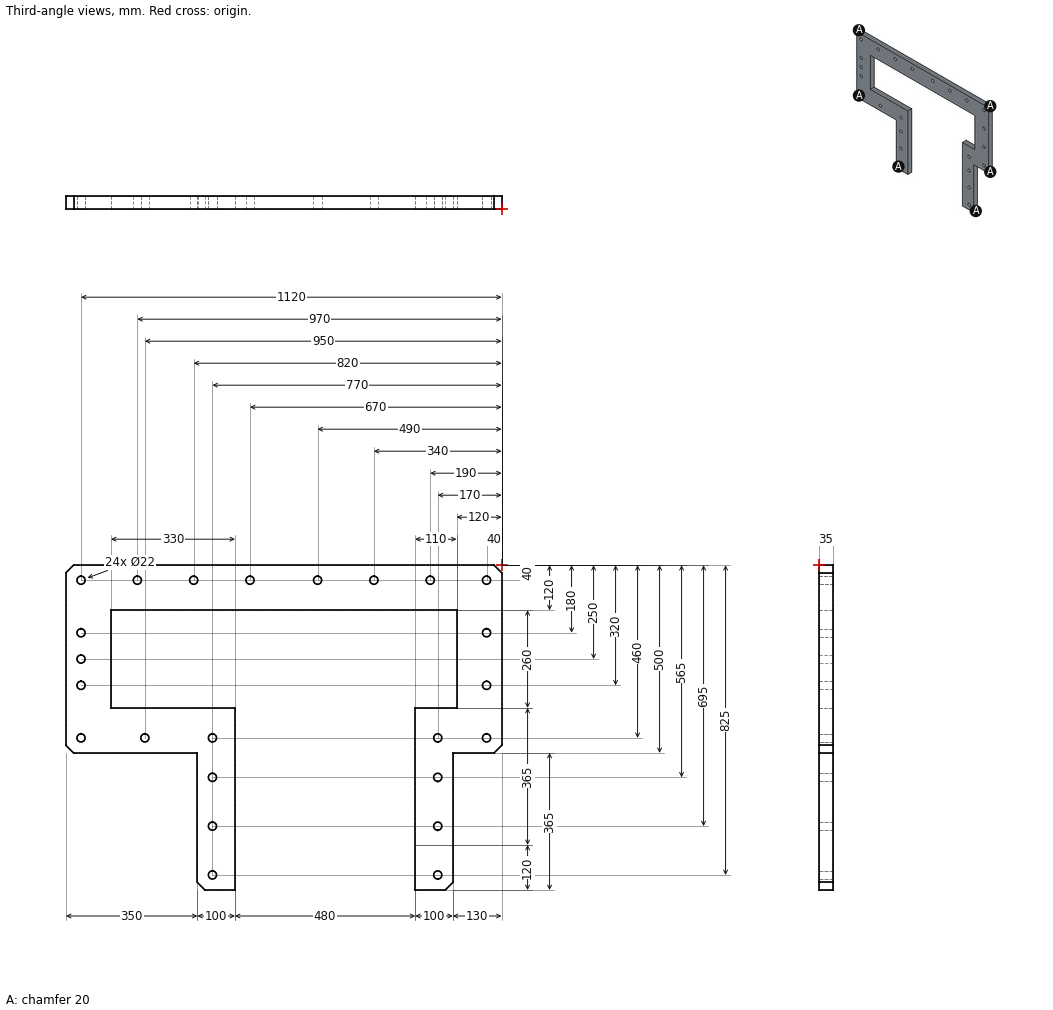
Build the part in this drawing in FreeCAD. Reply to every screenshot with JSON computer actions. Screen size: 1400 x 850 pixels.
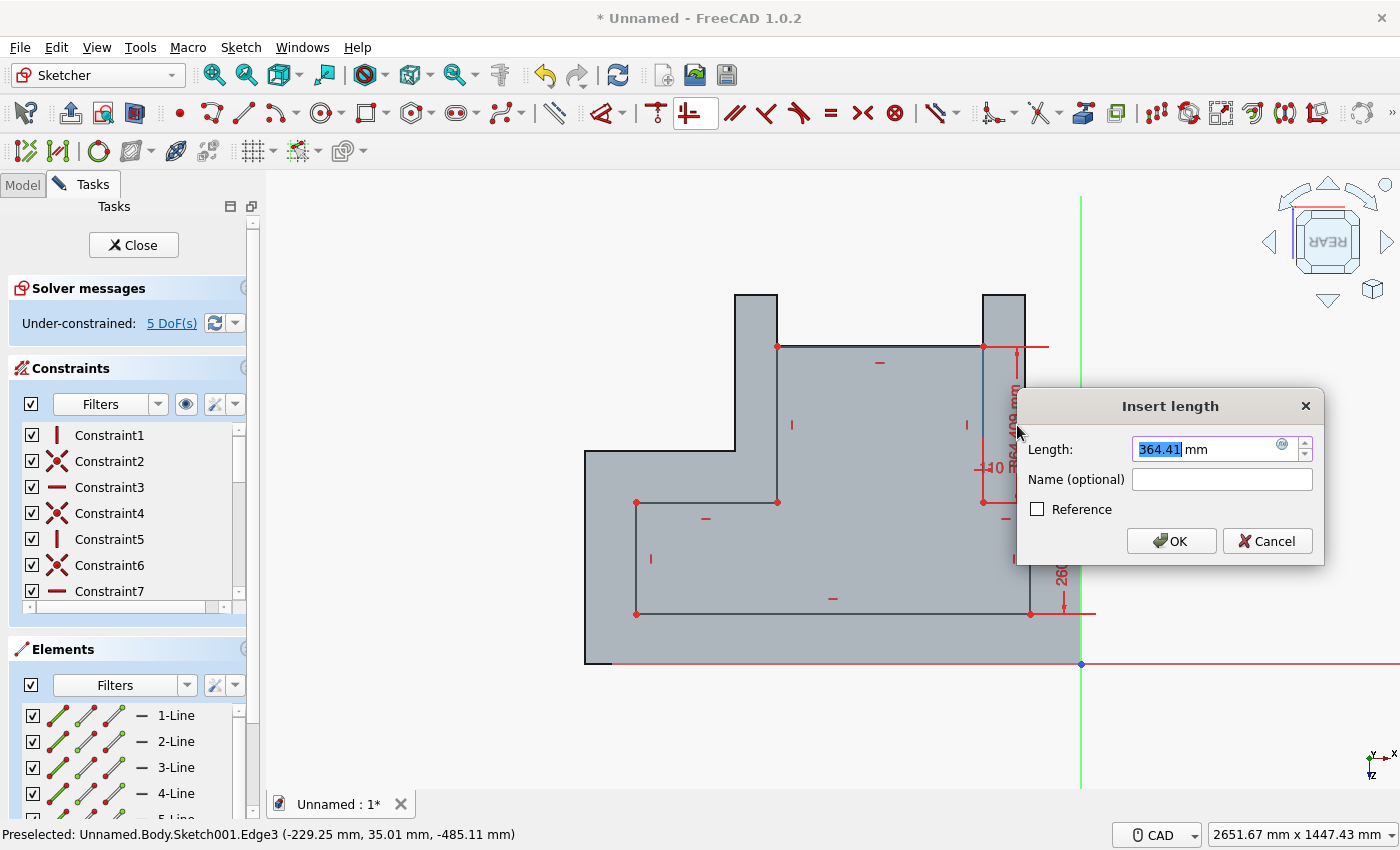
{"action": "type", "text": "365"}
{"action": "key", "text": "Return"}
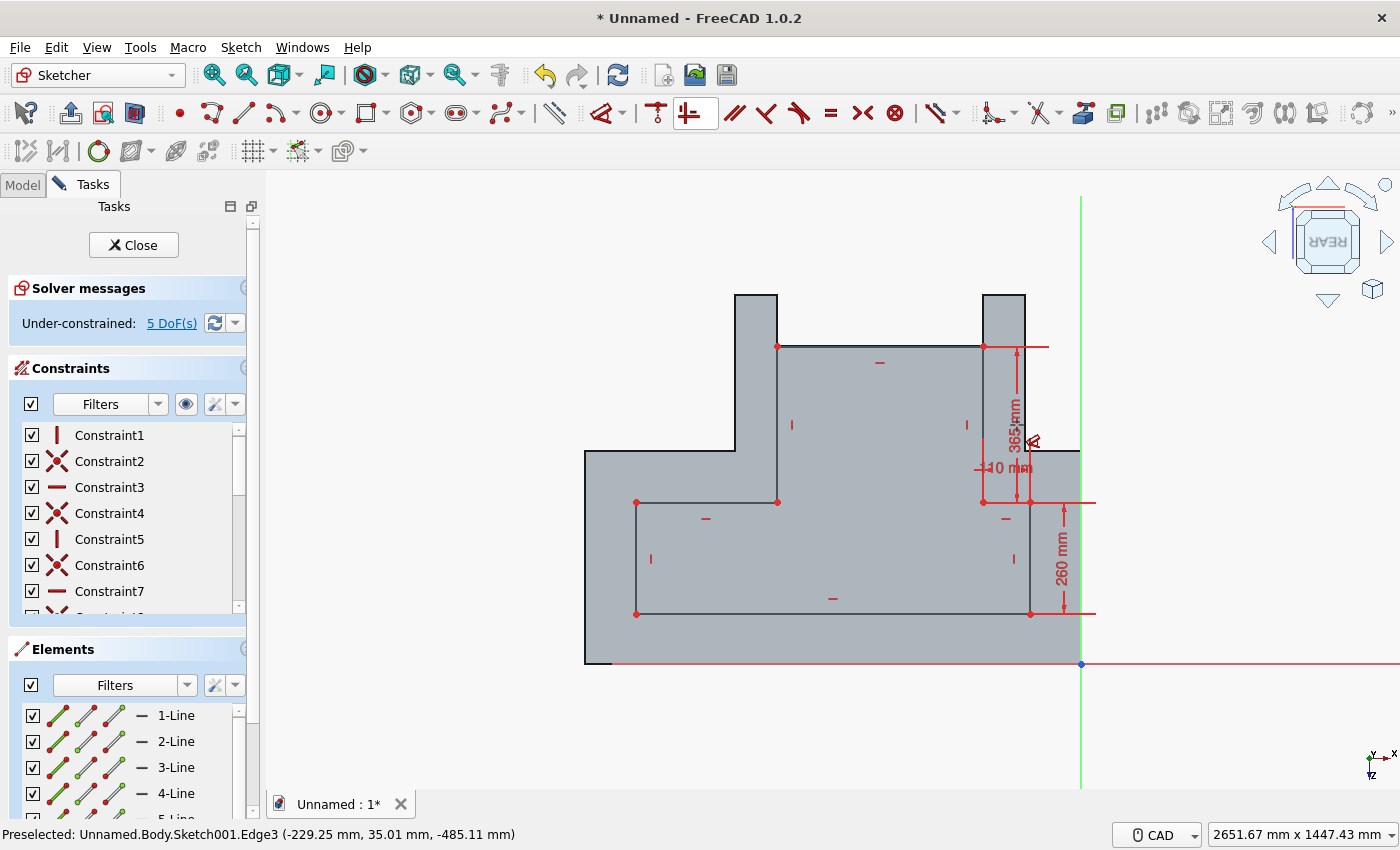
{"action": "left_click", "coordinate": [921, 347]}
{"action": "left_click", "coordinate": [880, 313]}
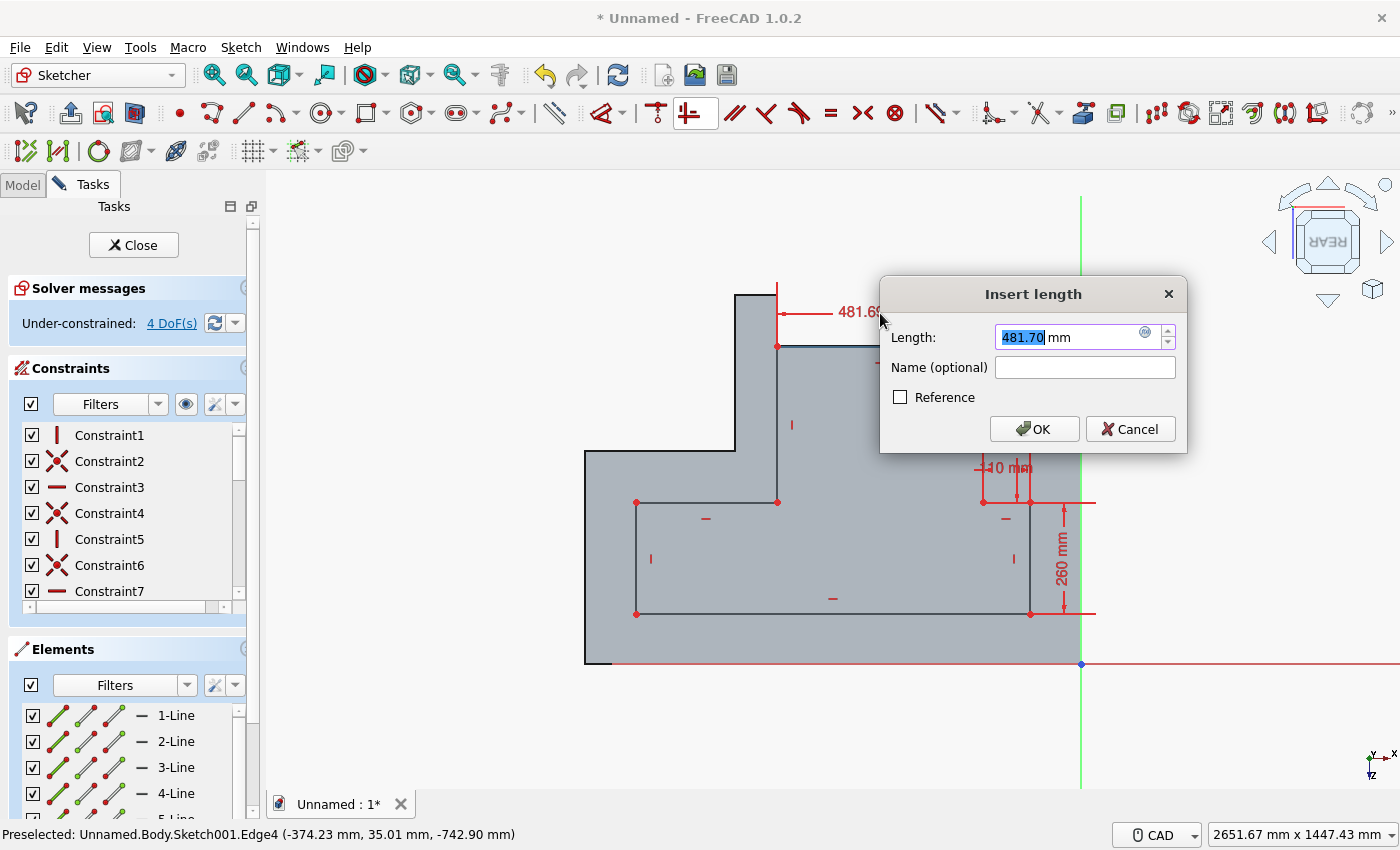
{"action": "type", "text": "480"}
{"action": "key", "text": "Return"}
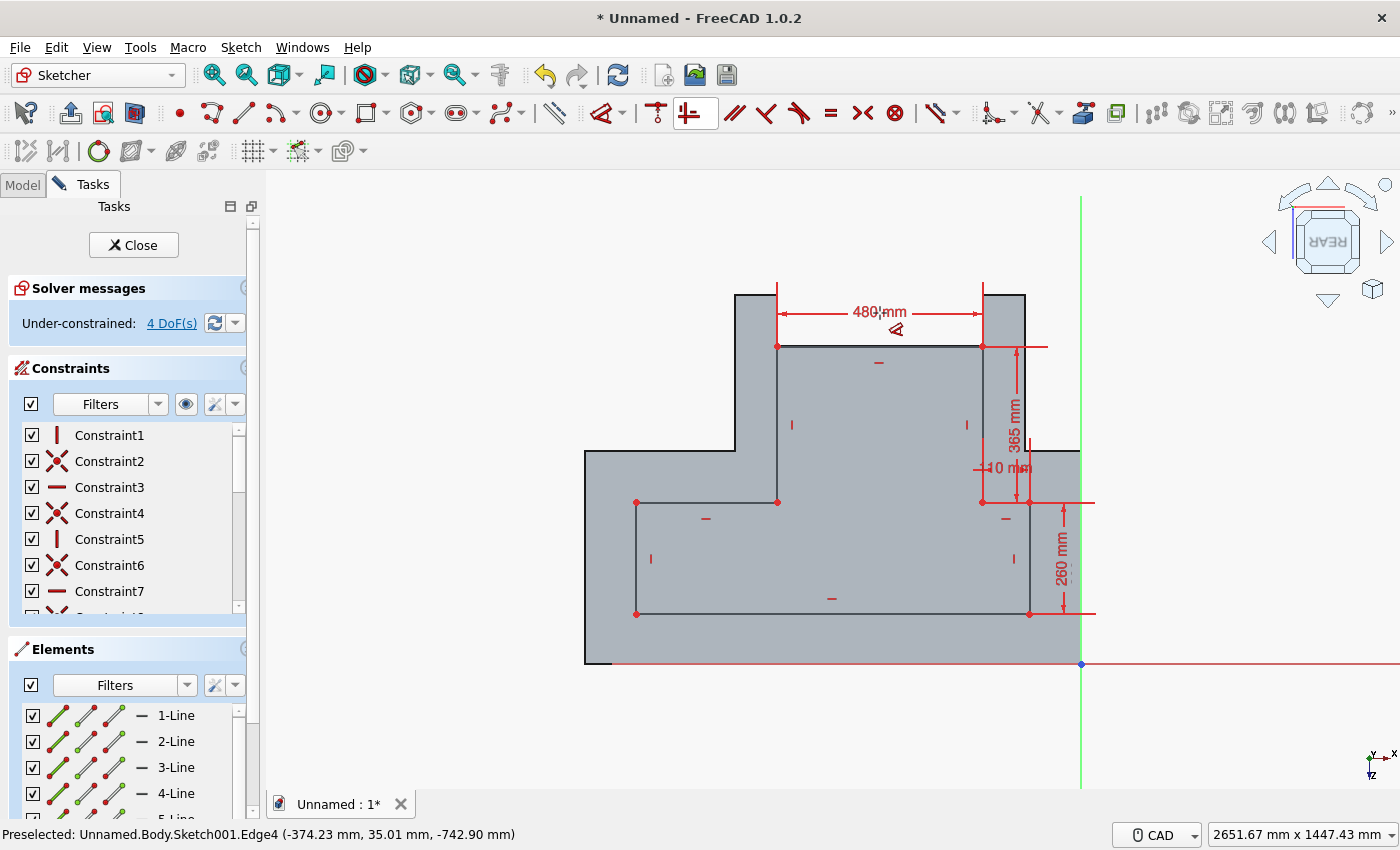
{"action": "left_click", "coordinate": [777, 394]}
{"action": "left_click", "coordinate": [743, 425]}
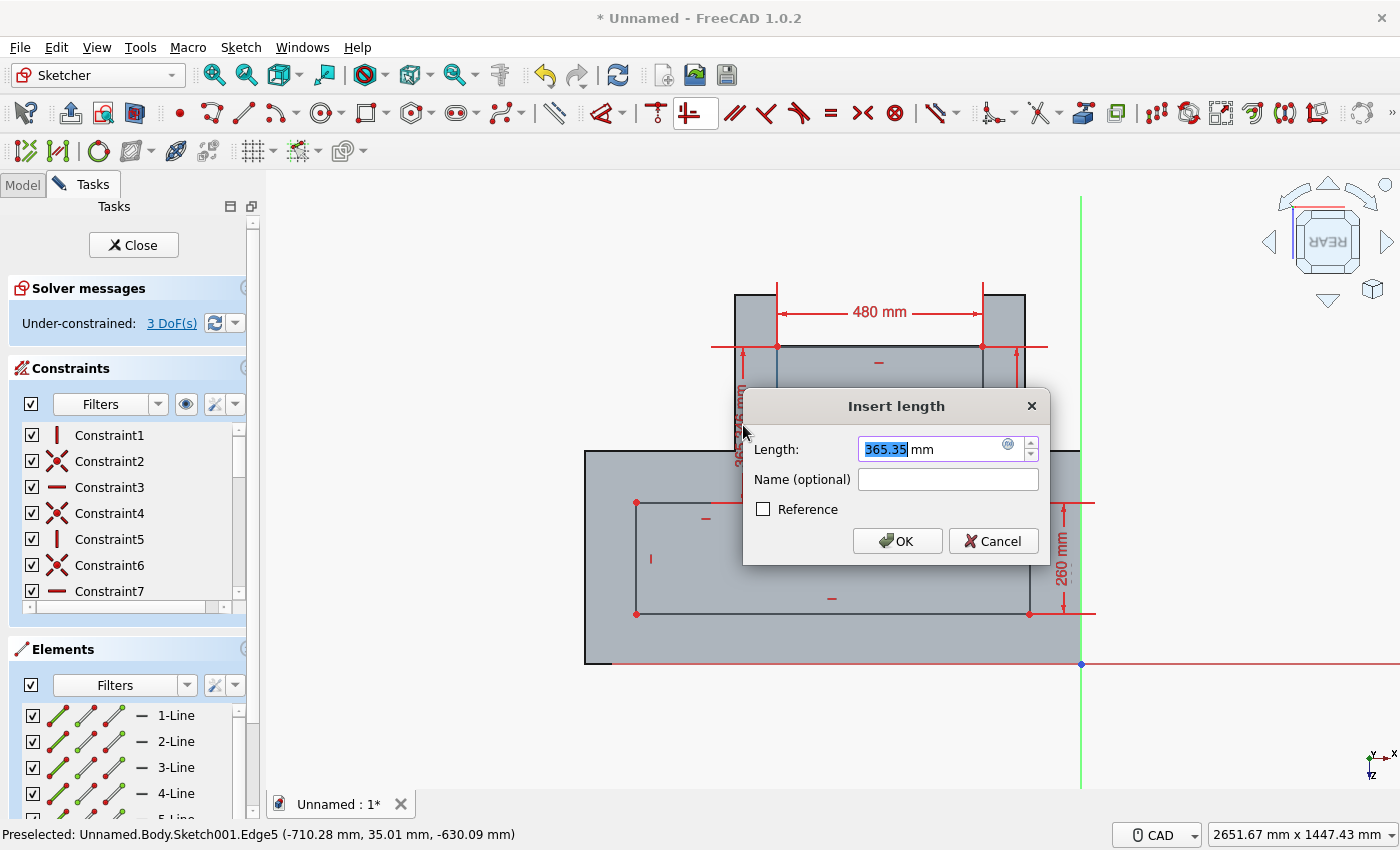
{"action": "type", "text": "365"}
{"action": "key", "text": "Return"}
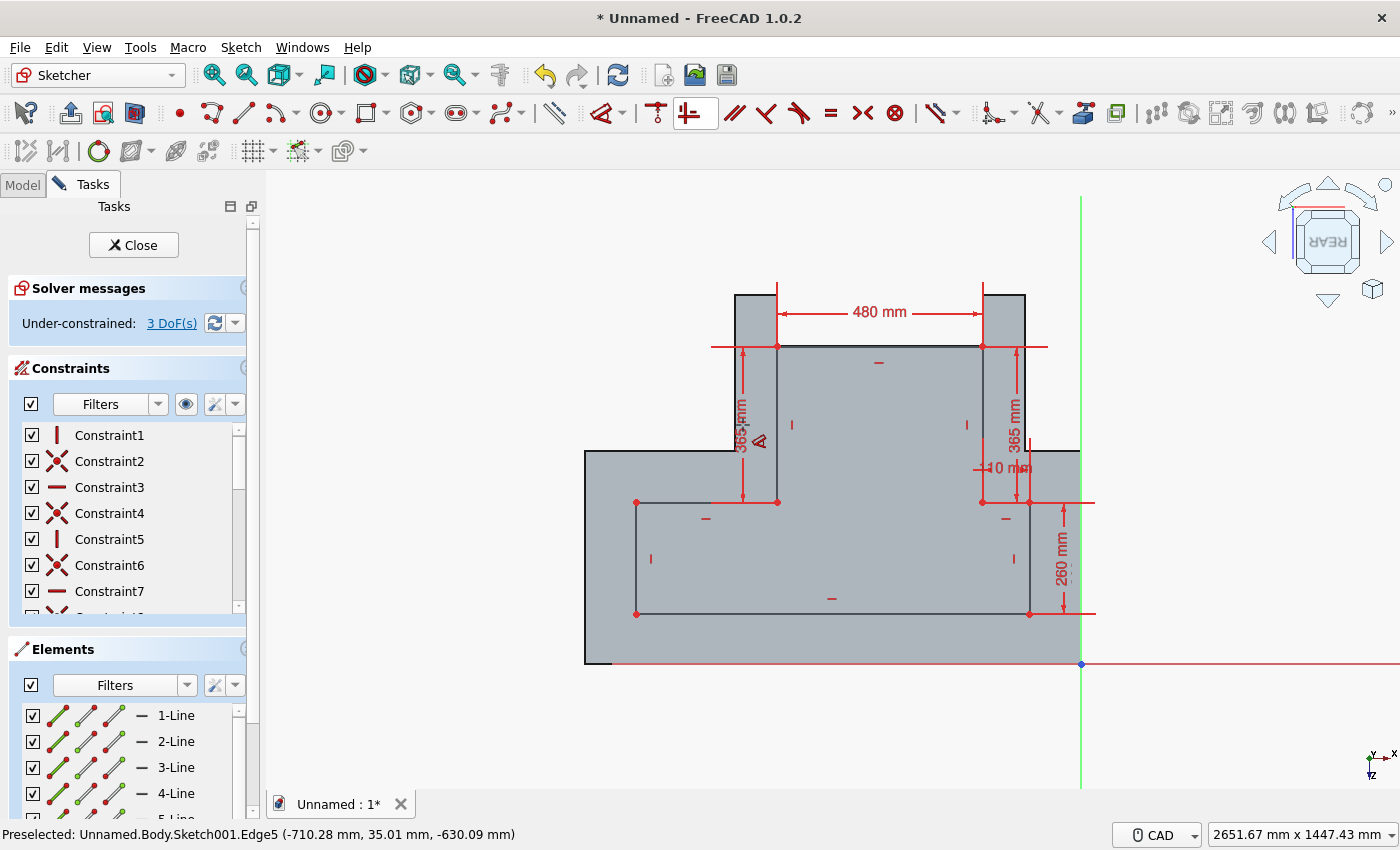
{"action": "left_click", "coordinate": [735, 503]}
{"action": "left_click", "coordinate": [707, 469]}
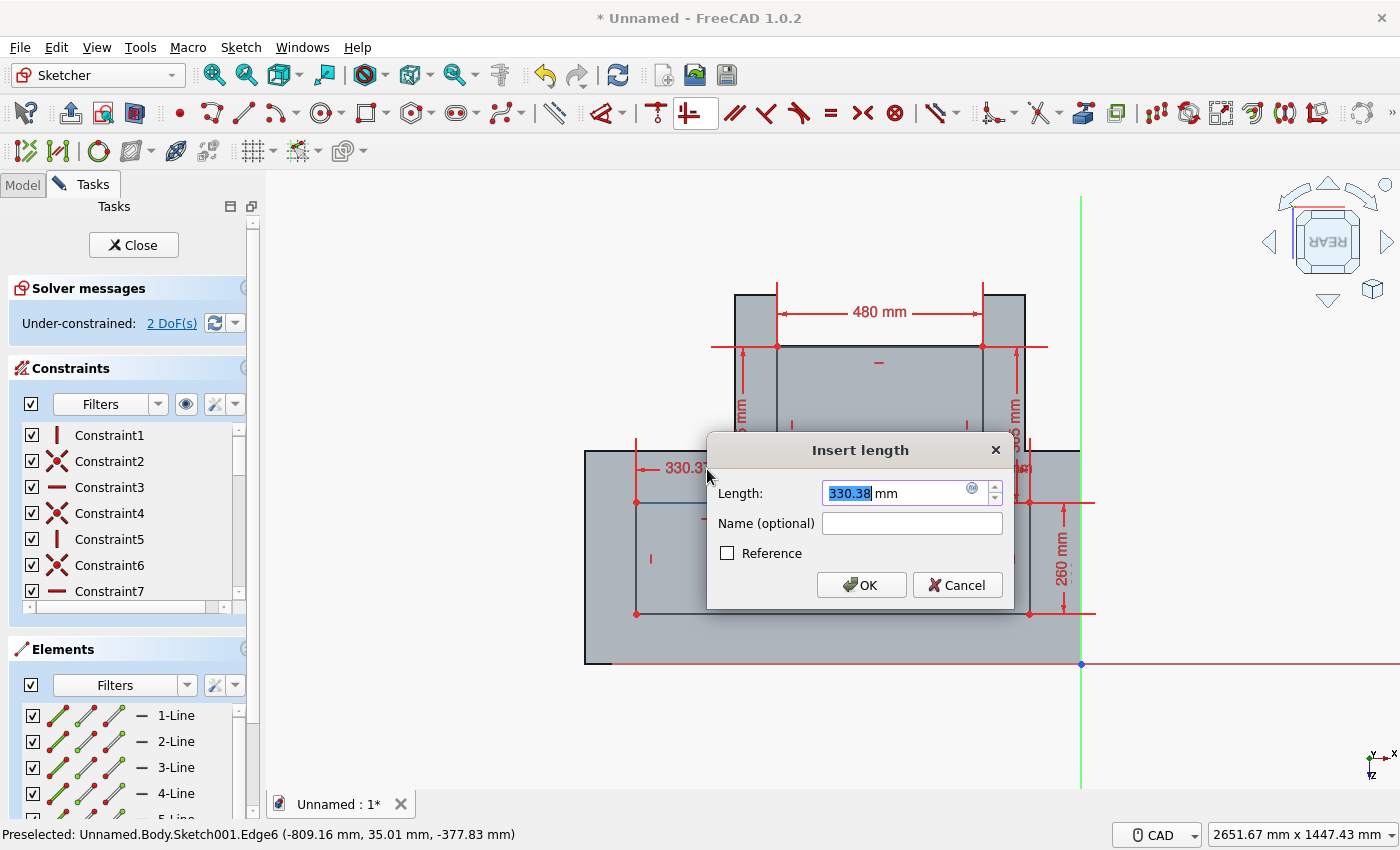
{"action": "type", "text": "330"}
{"action": "key", "text": "Return"}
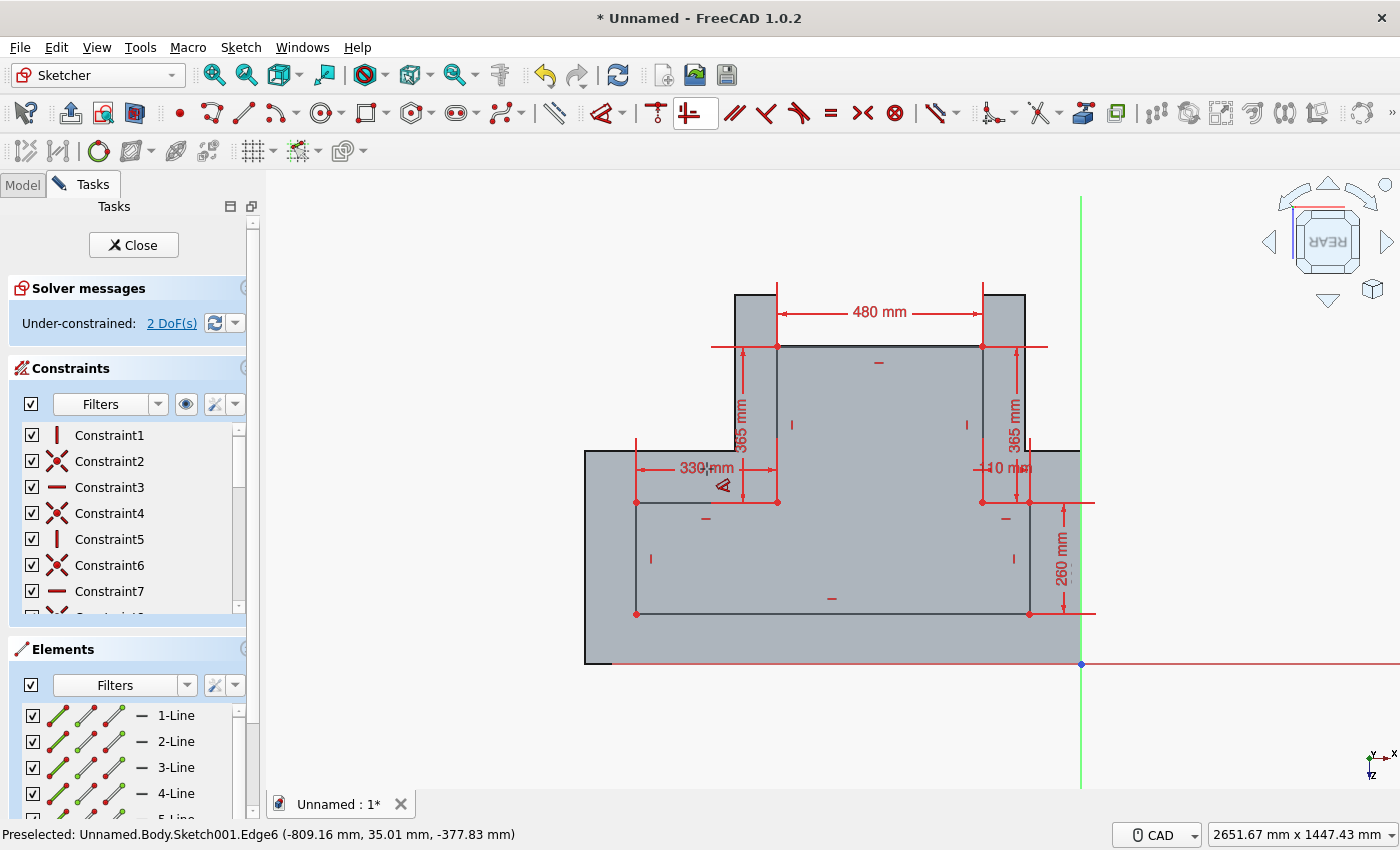
{"action": "left_click", "coordinate": [1030, 614]}
{"action": "left_click", "coordinate": [1055, 698]}